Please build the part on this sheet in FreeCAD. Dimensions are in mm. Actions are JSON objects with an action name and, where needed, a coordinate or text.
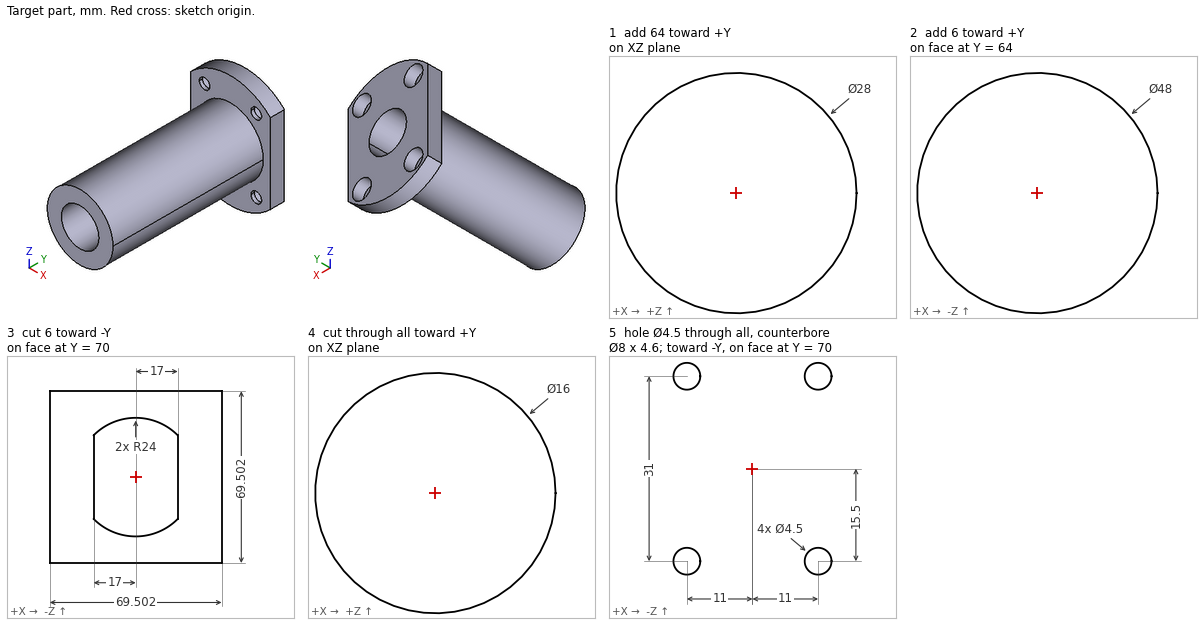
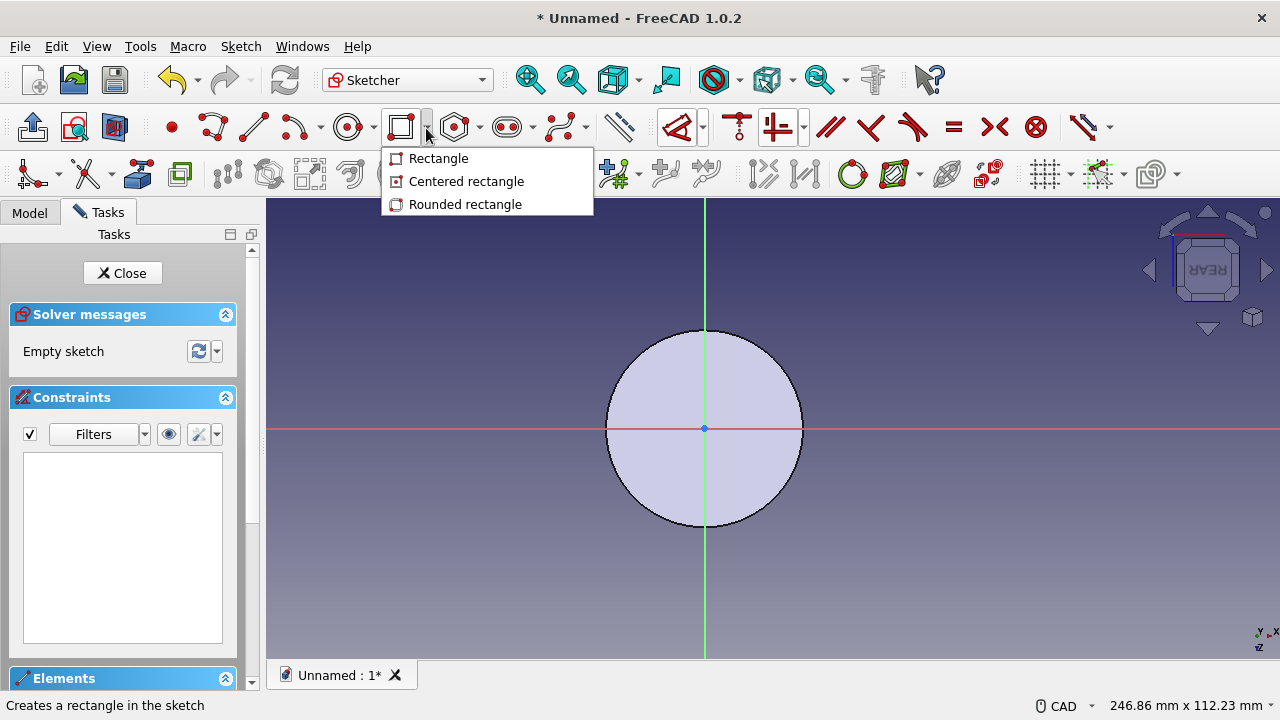
{"action": "left_click", "coordinate": [488, 182]}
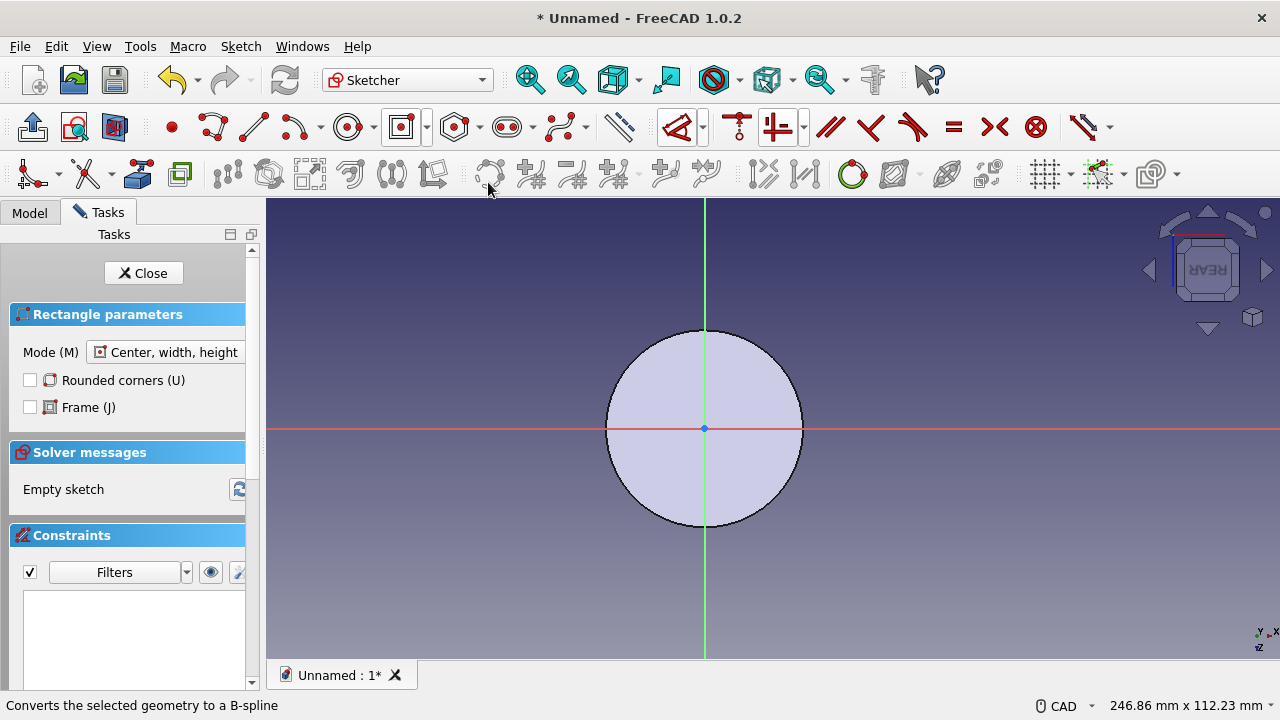
{"action": "left_click", "coordinate": [705, 429]}
{"action": "left_click", "coordinate": [847, 286]}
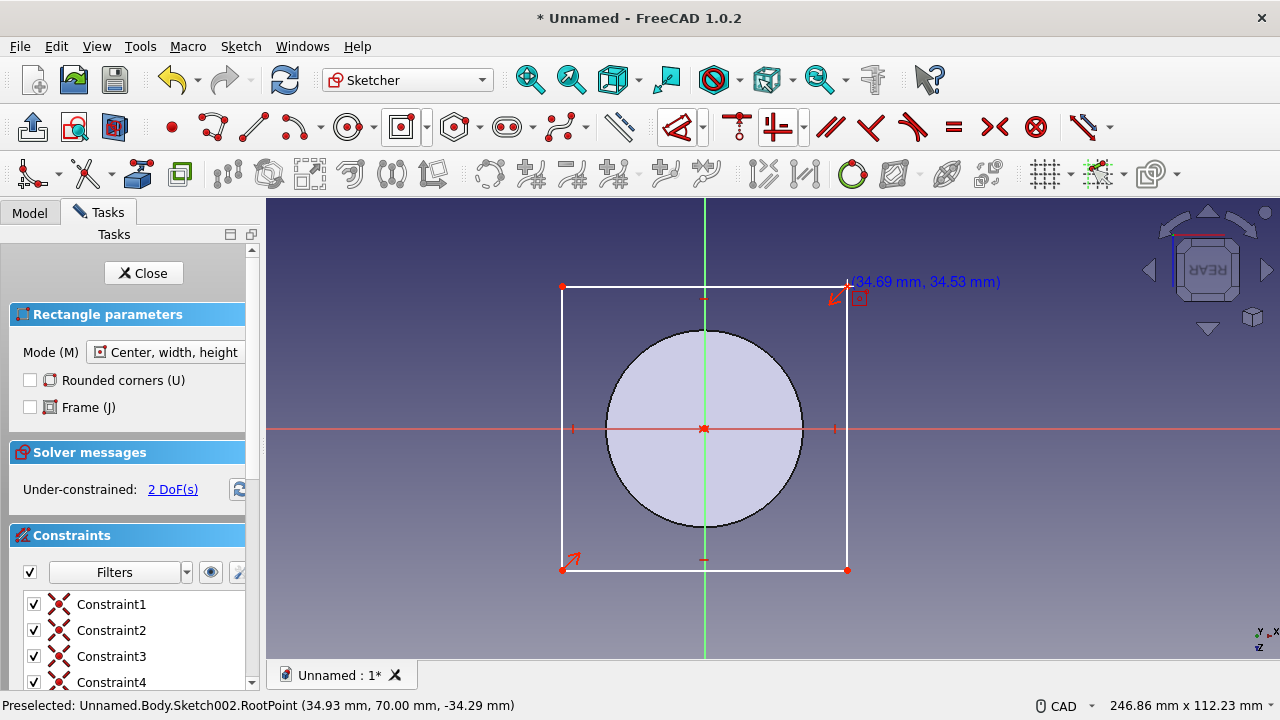
{"action": "left_click", "coordinate": [254, 128]}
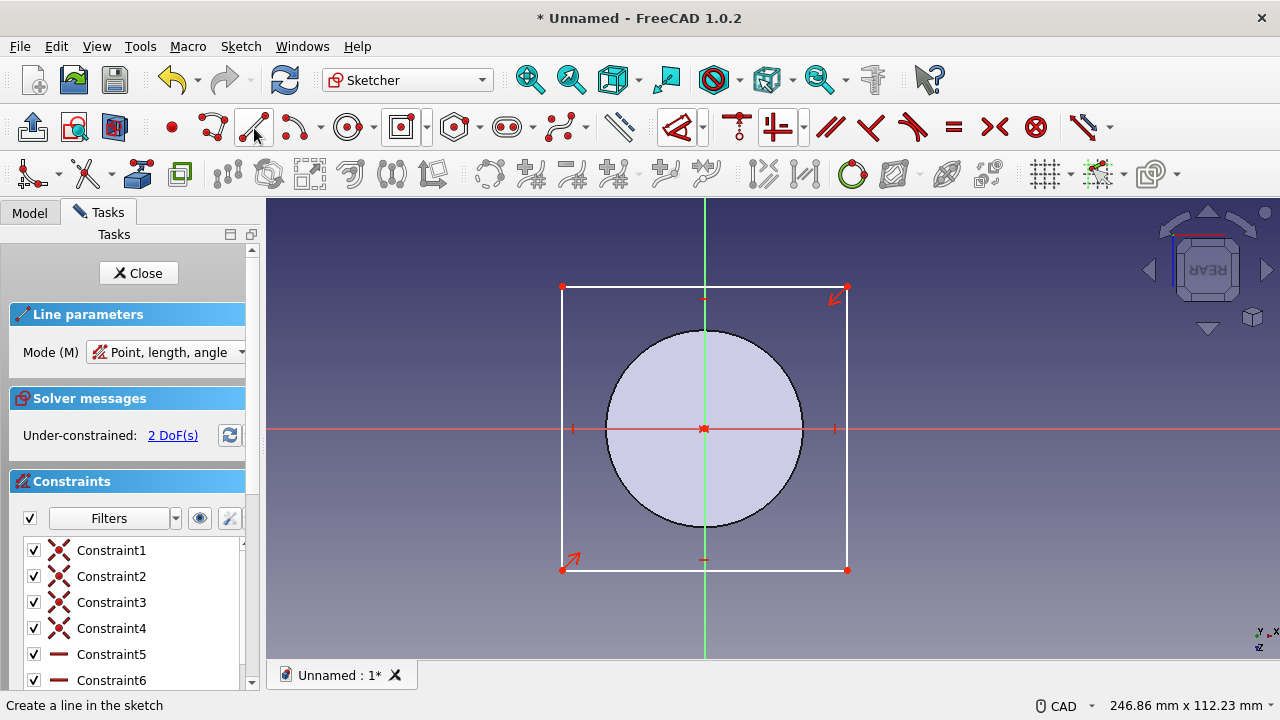
{"action": "left_click", "coordinate": [635, 498]}
{"action": "left_click", "coordinate": [635, 359]}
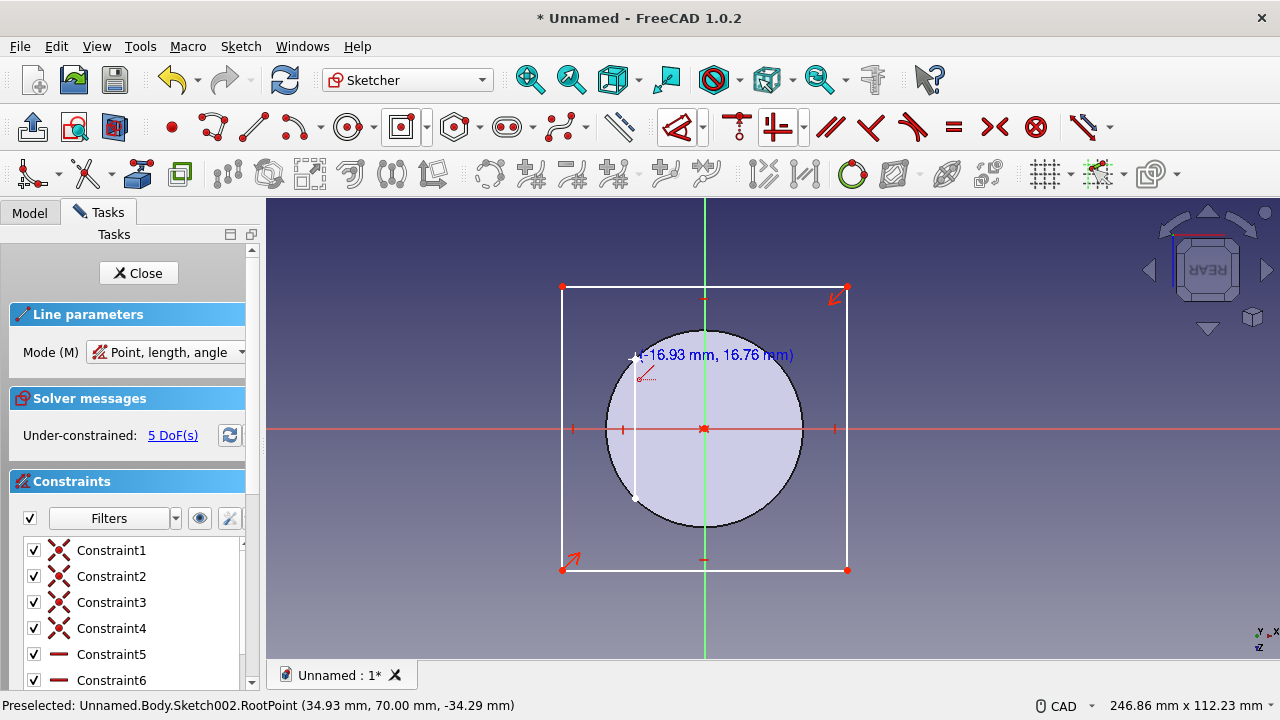
{"action": "left_click", "coordinate": [774, 359]}
{"action": "left_click", "coordinate": [774, 498]}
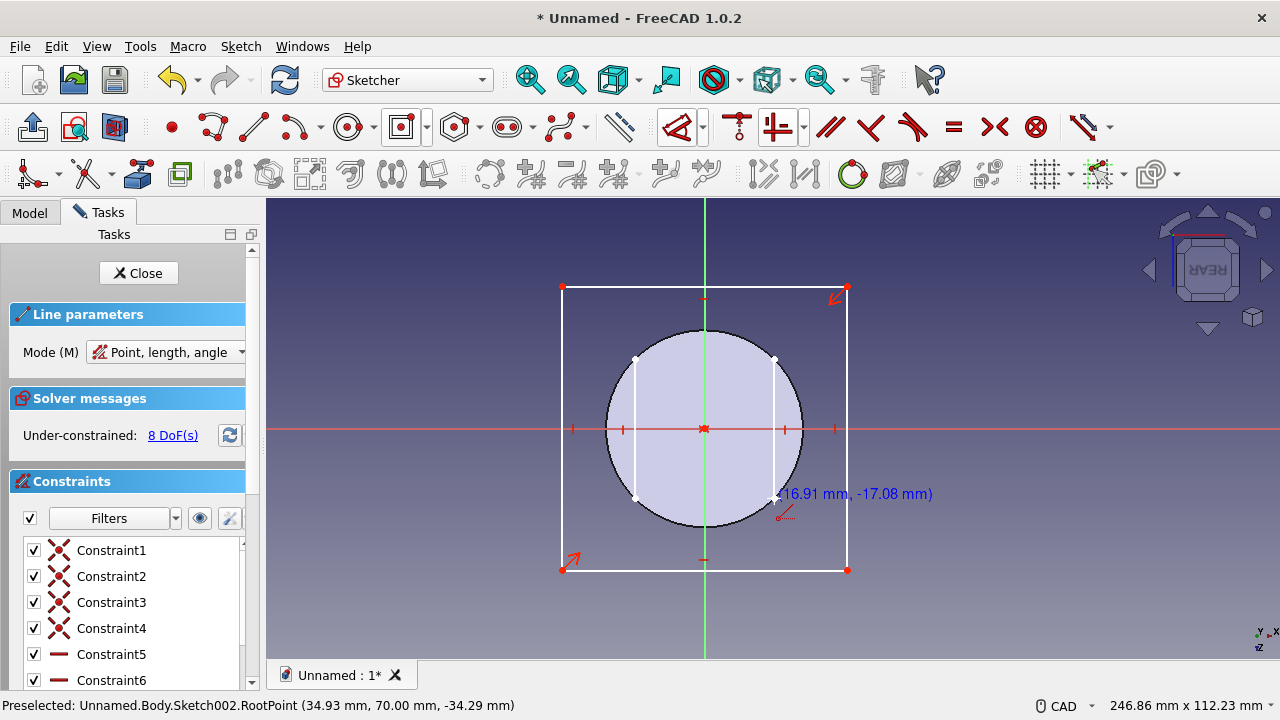
{"action": "left_click", "coordinate": [320, 128]}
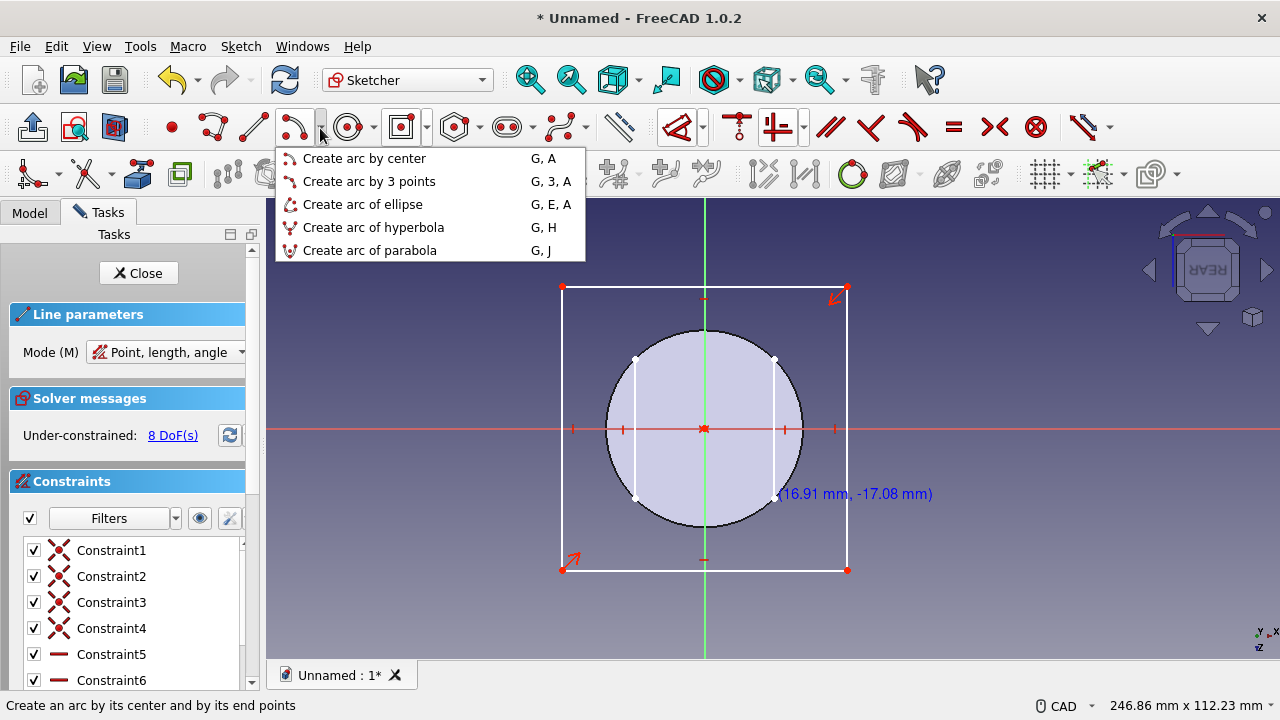
{"action": "left_click", "coordinate": [430, 182]}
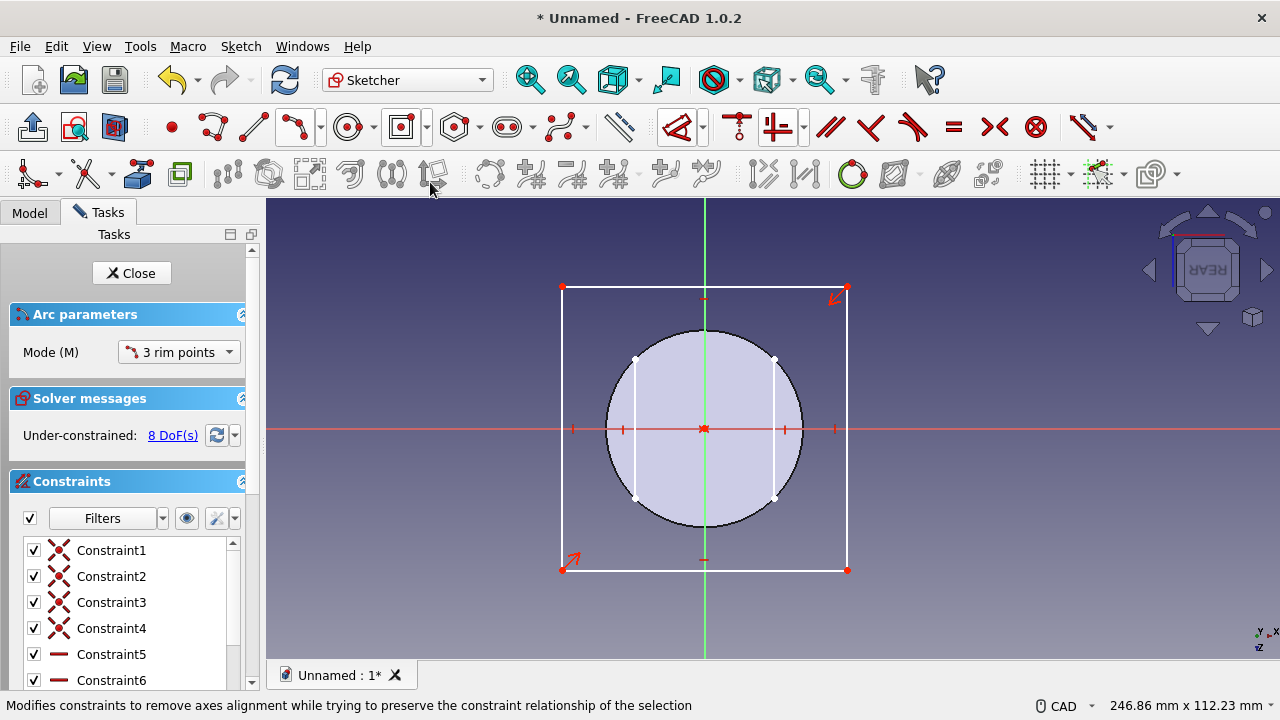
{"action": "left_click", "coordinate": [635, 360]}
{"action": "left_click", "coordinate": [774, 360]}
{"action": "left_click", "coordinate": [720, 331]}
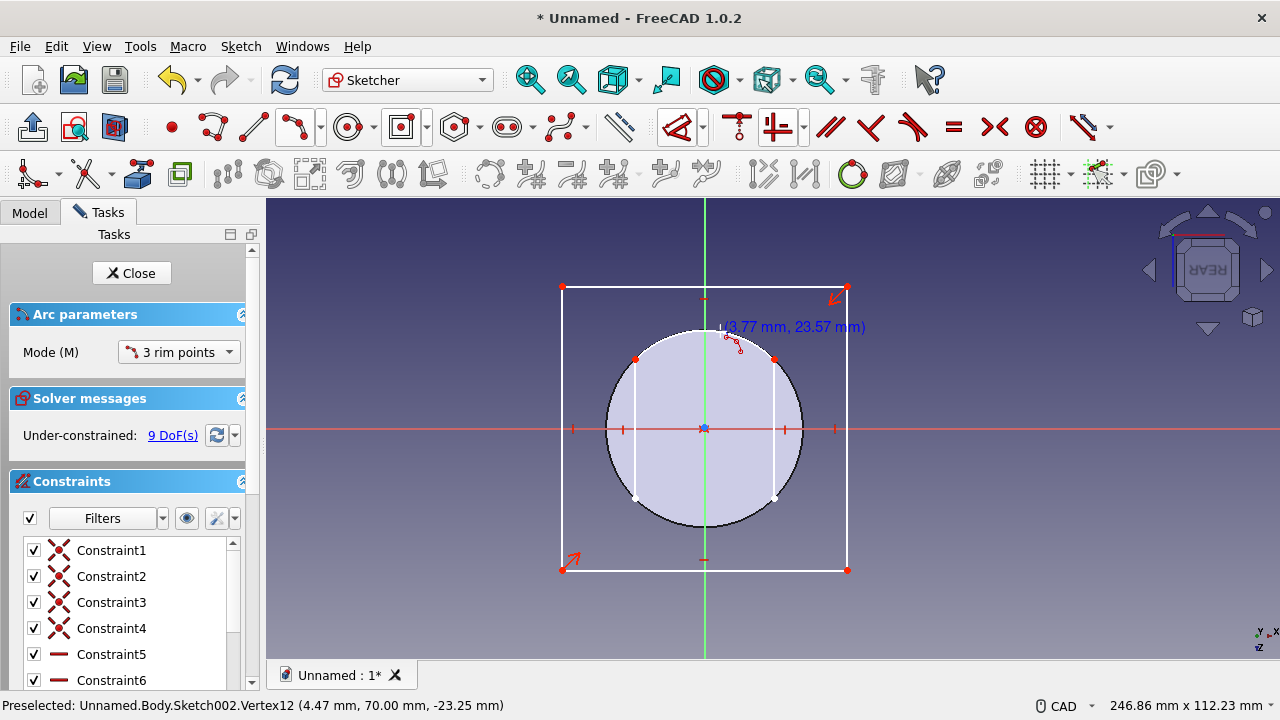
{"action": "left_click", "coordinate": [774, 499]}
{"action": "left_click", "coordinate": [635, 499]}
{"action": "left_click", "coordinate": [689, 526]}
{"action": "key", "text": "Escape"}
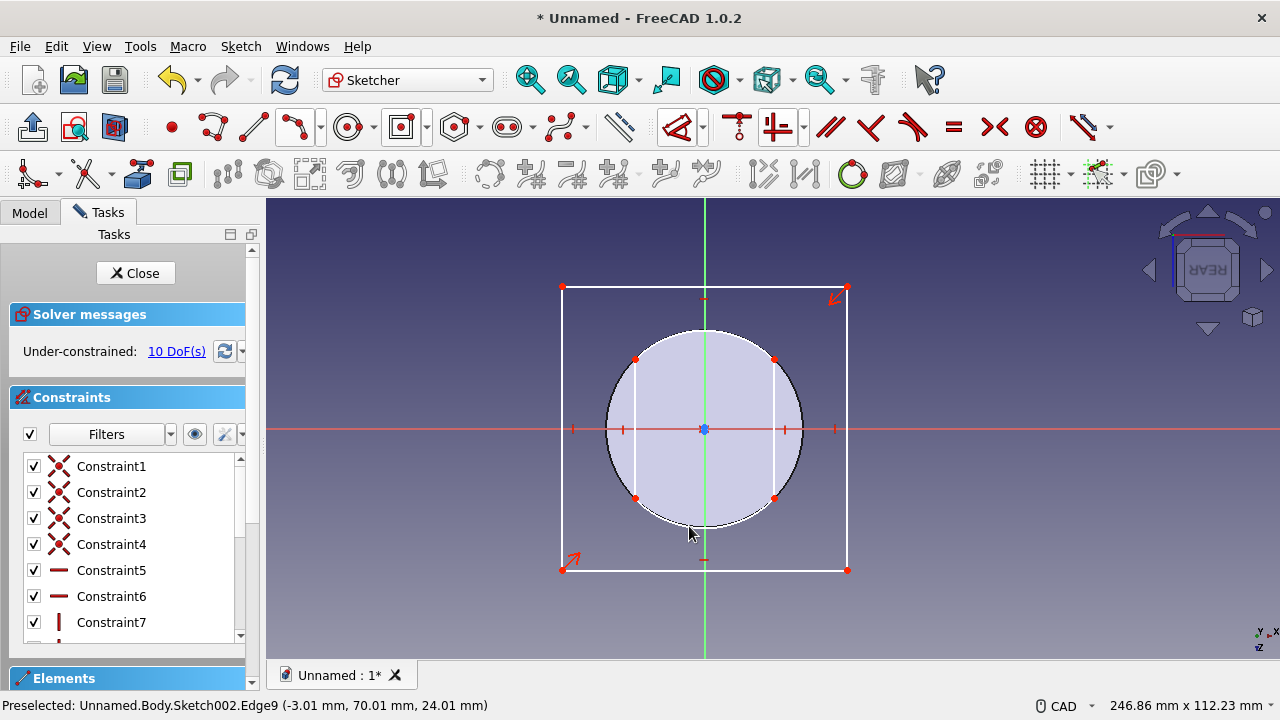
{"action": "left_click", "coordinate": [735, 336]}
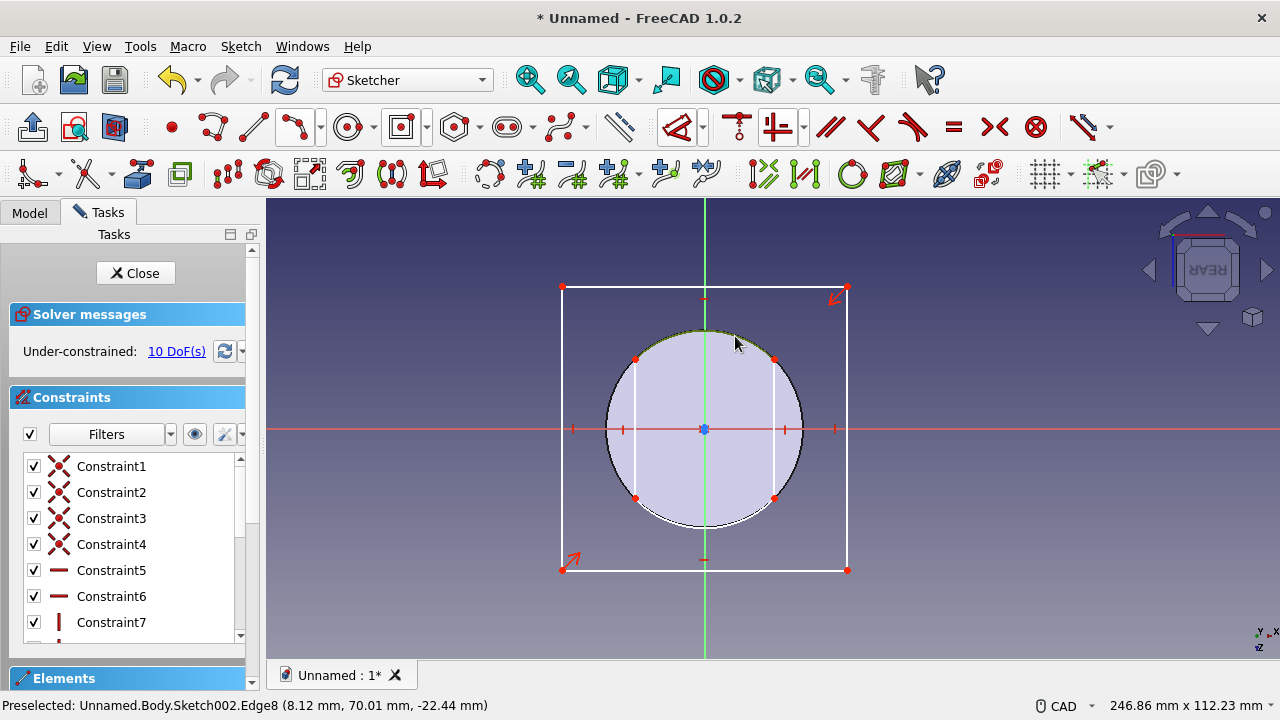
{"action": "left_click", "coordinate": [674, 523]}